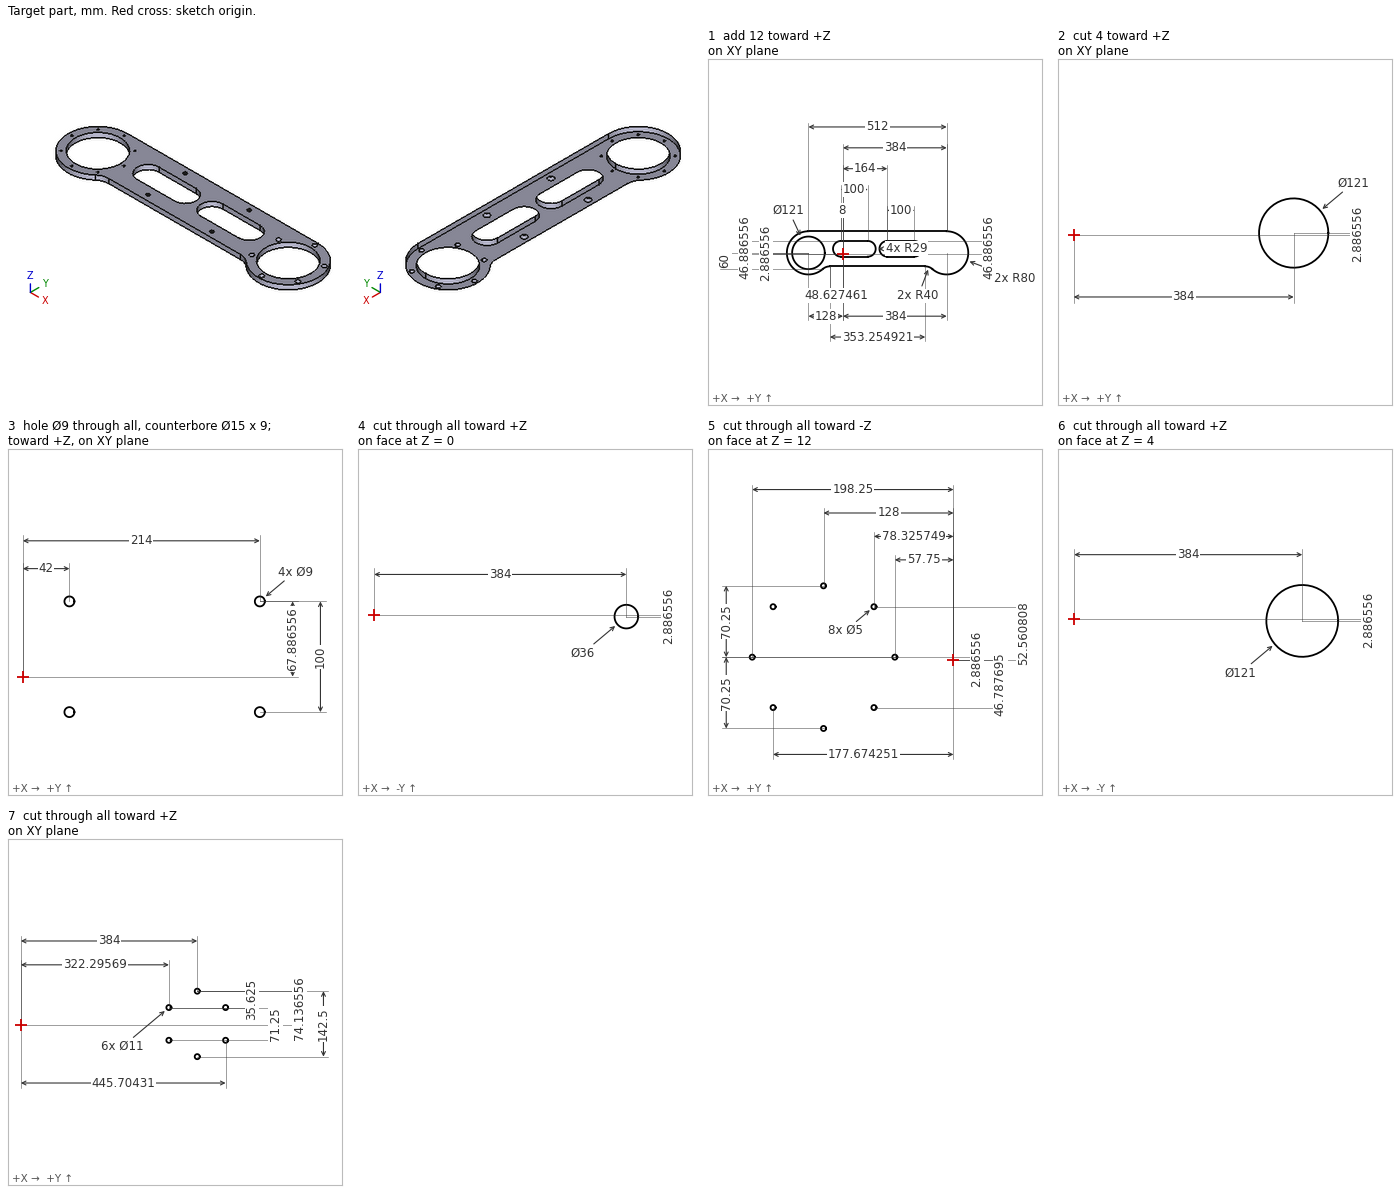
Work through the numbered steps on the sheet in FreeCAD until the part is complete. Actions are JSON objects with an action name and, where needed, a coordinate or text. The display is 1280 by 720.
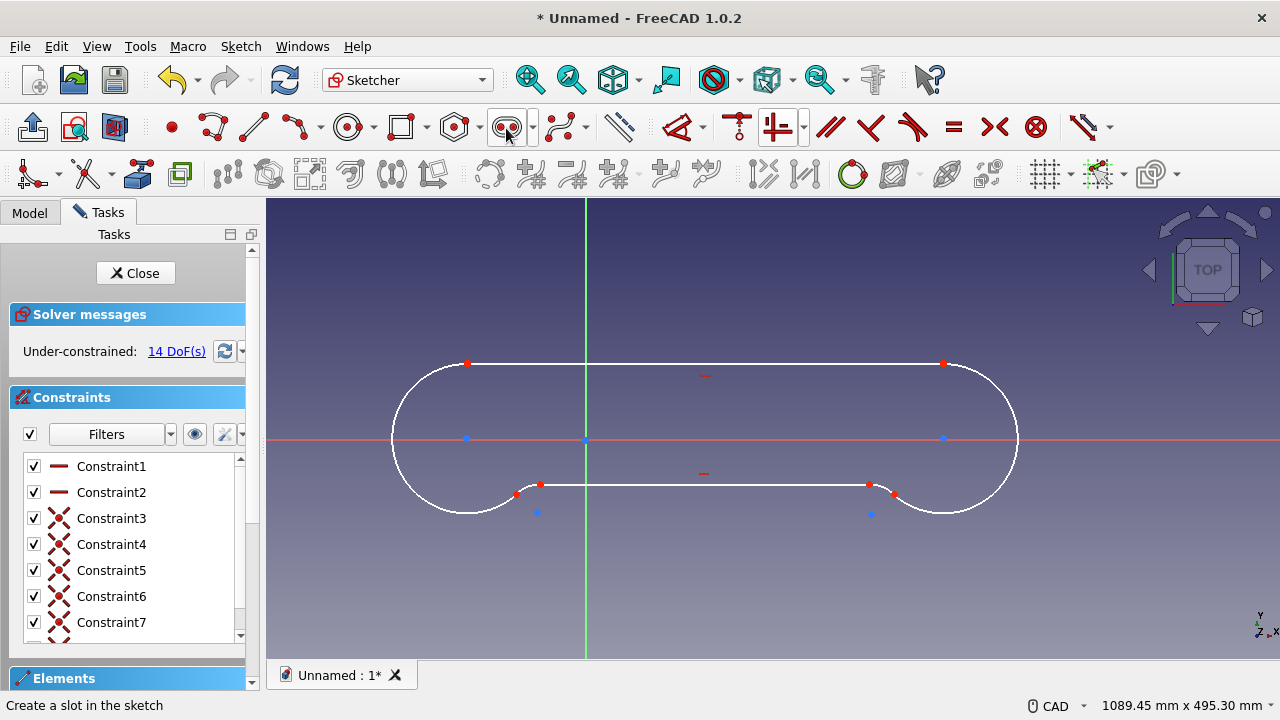
{"action": "left_click", "coordinate": [738, 424]}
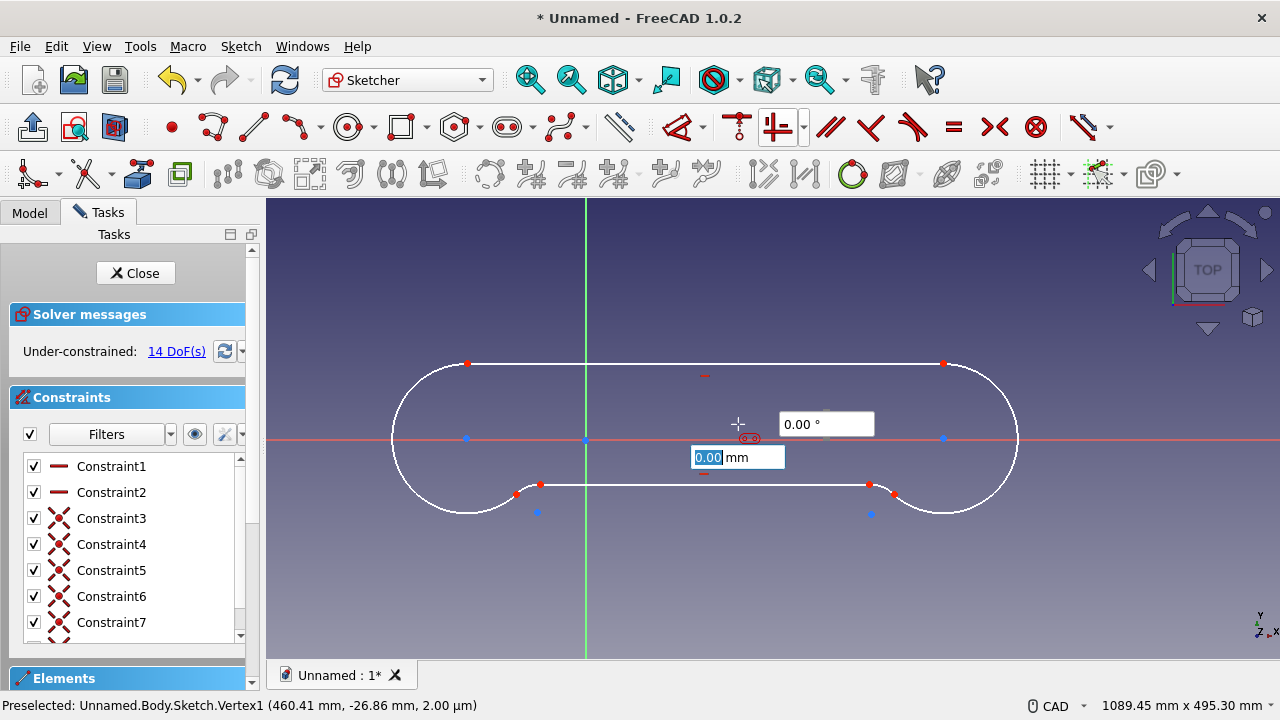
{"action": "left_click", "coordinate": [831, 424]}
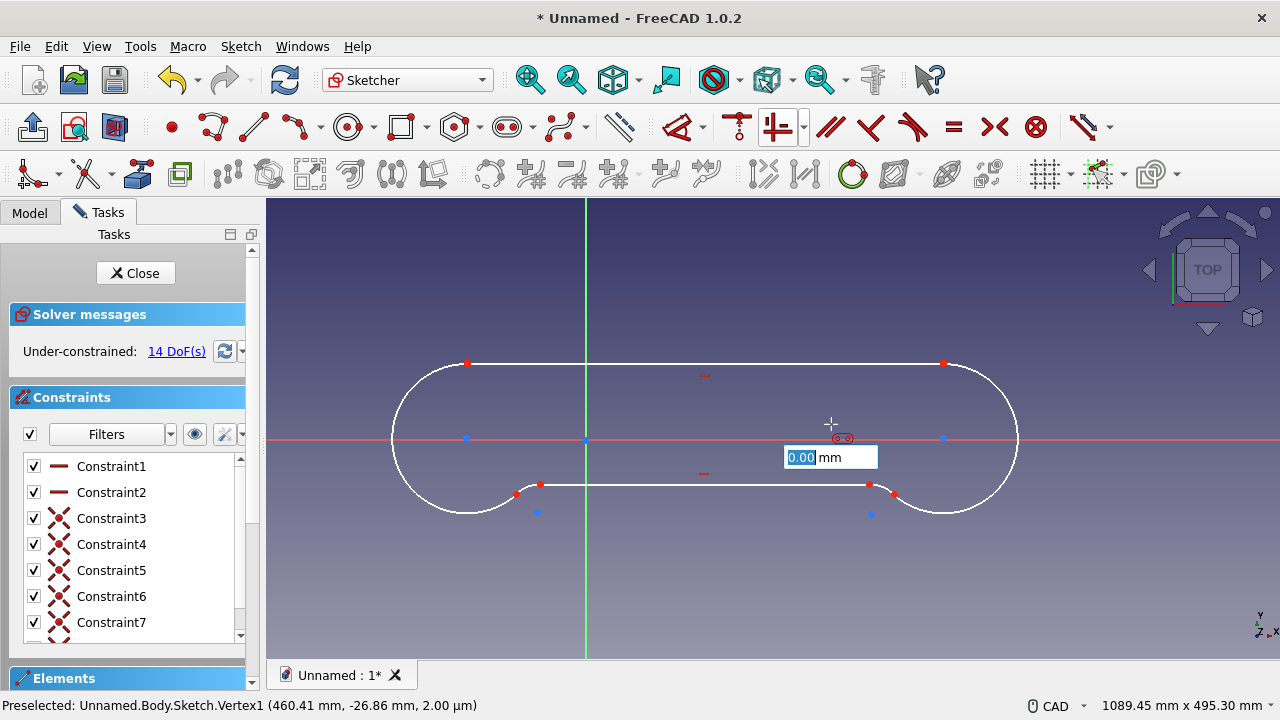
{"action": "left_click", "coordinate": [785, 397]}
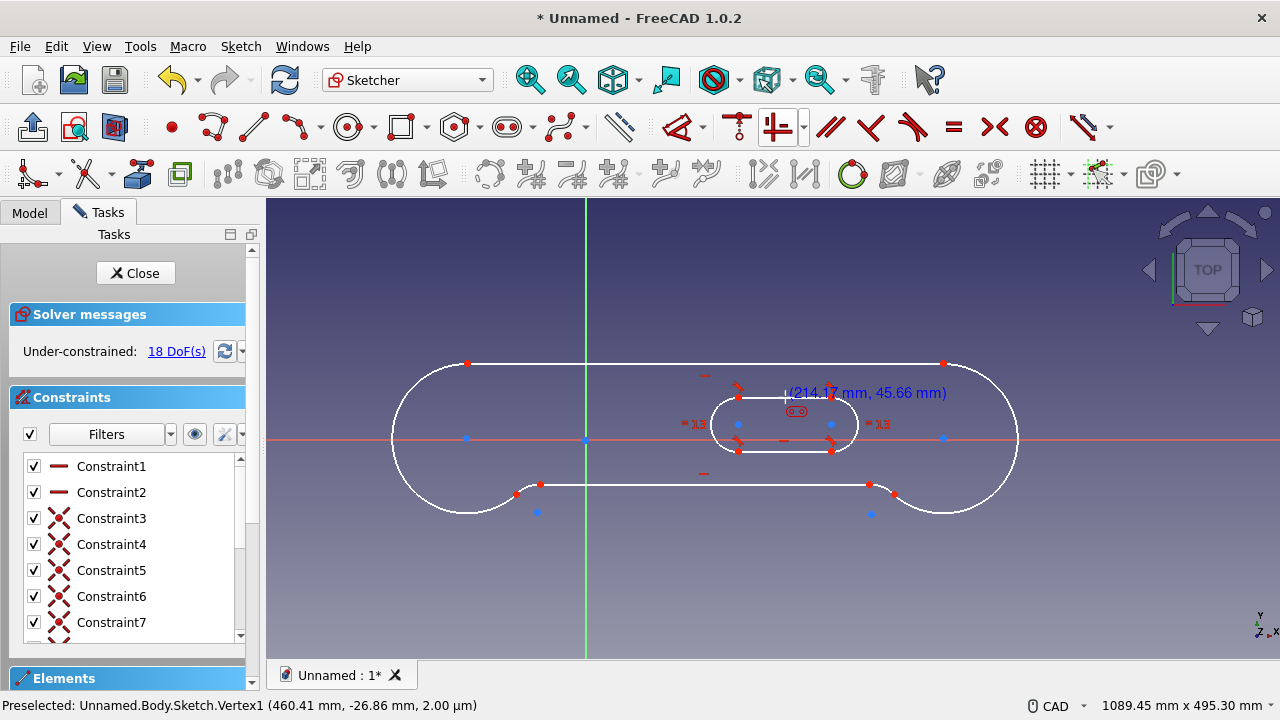
{"action": "scroll", "coordinate": [578, 424], "scroll_direction": "up", "scroll_amount": 4}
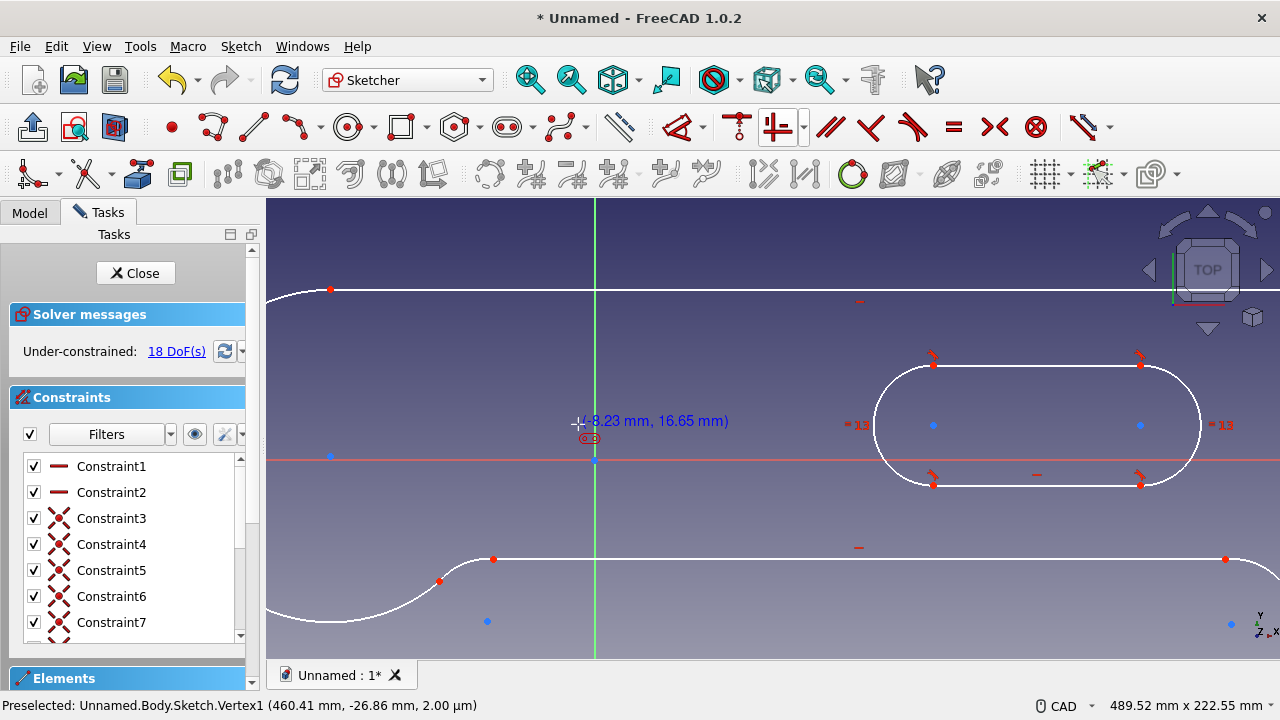
{"action": "left_click", "coordinate": [578, 423]}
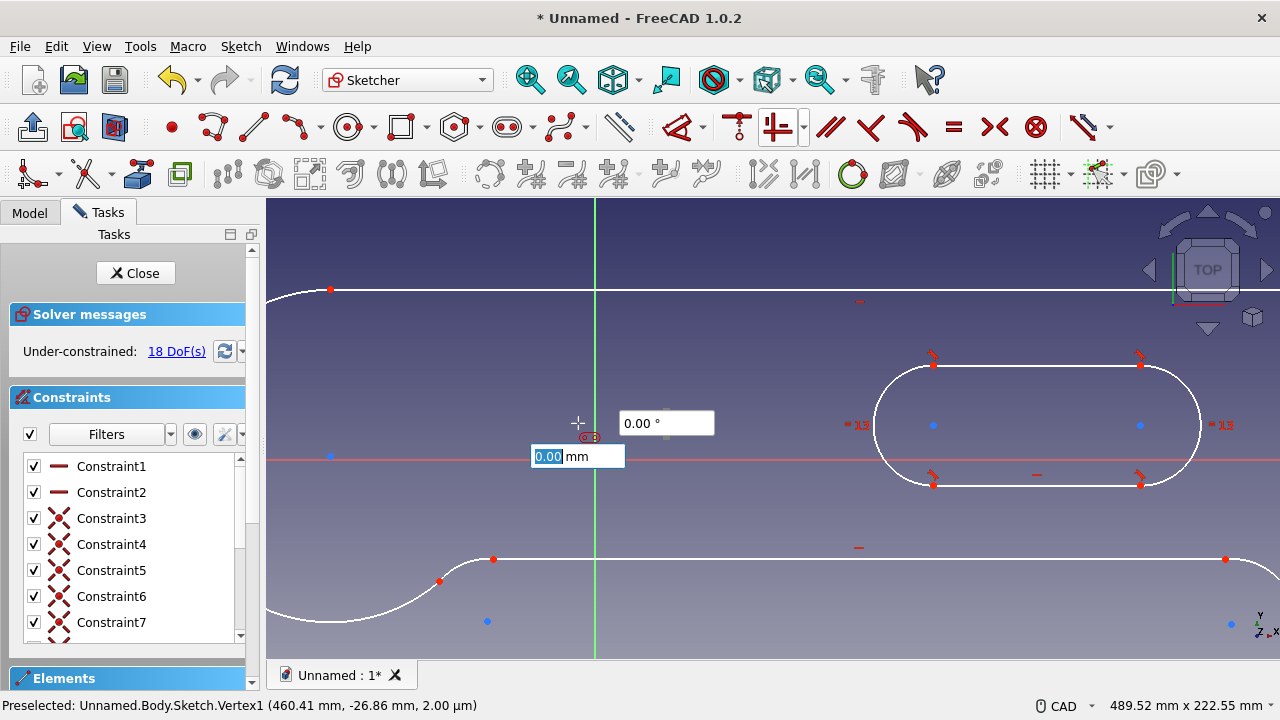
{"action": "left_click", "coordinate": [785, 423]}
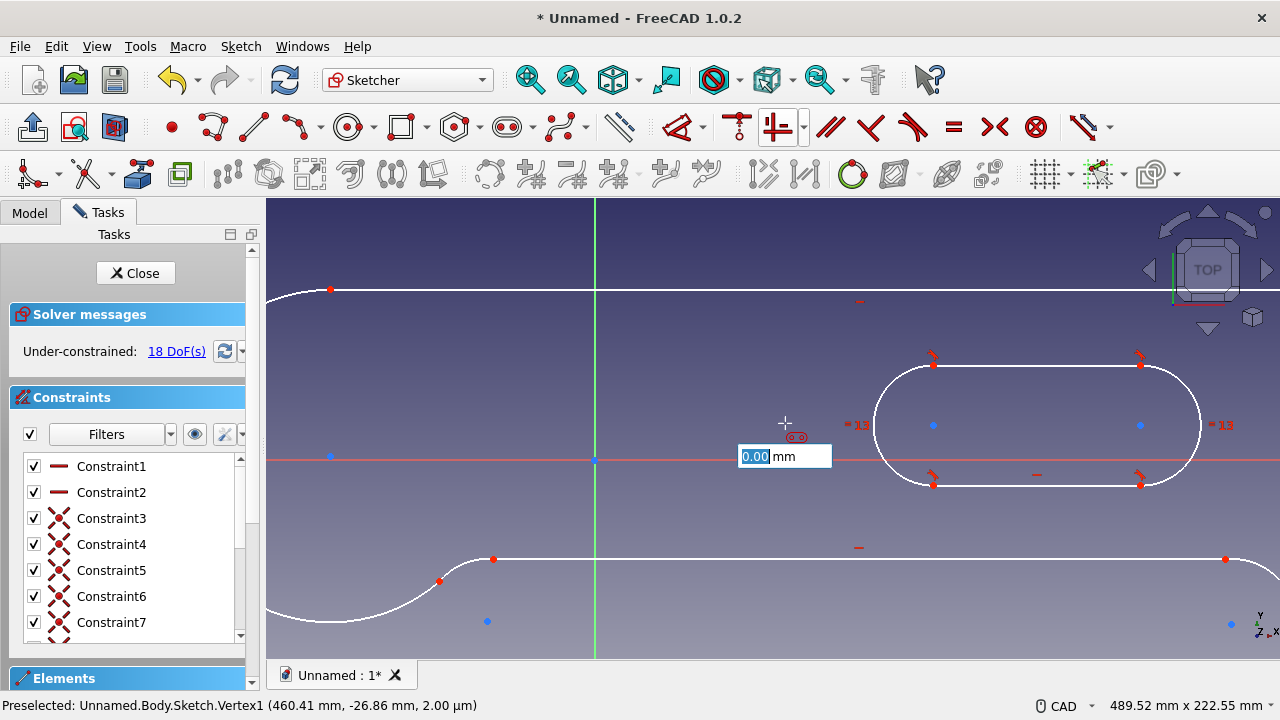
{"action": "left_click", "coordinate": [682, 363]}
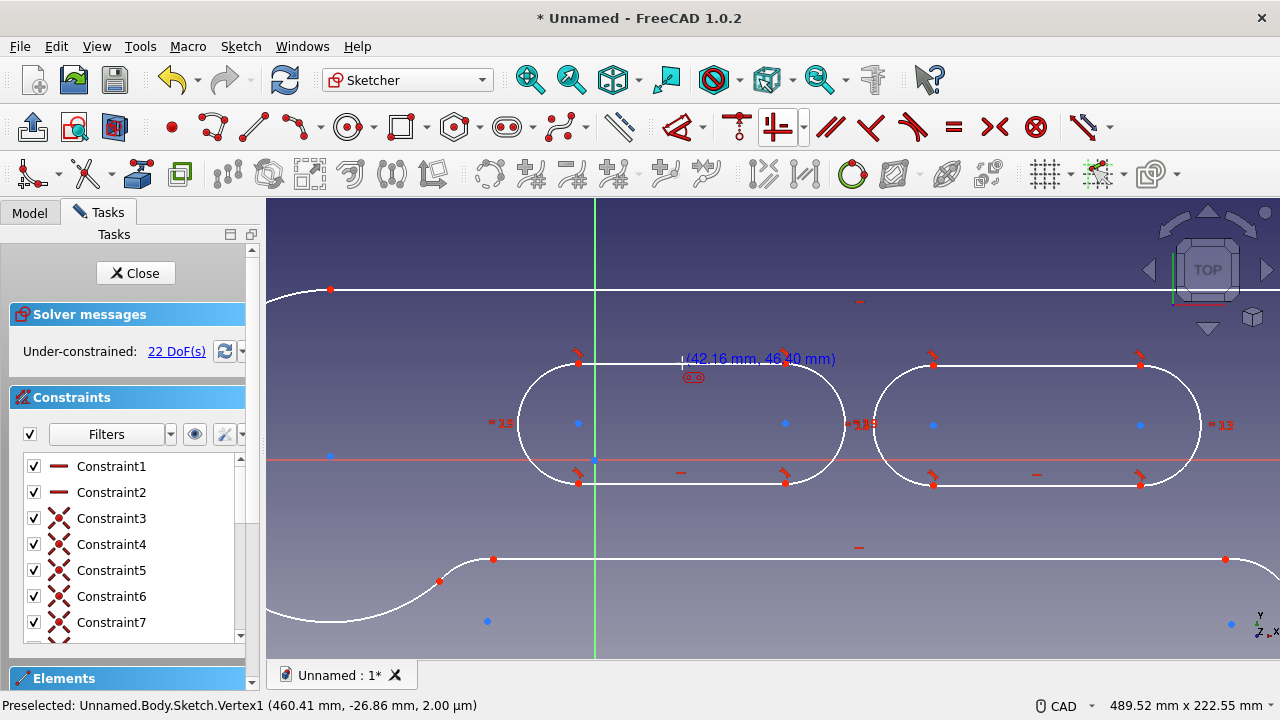
{"action": "left_click", "coordinate": [348, 128]}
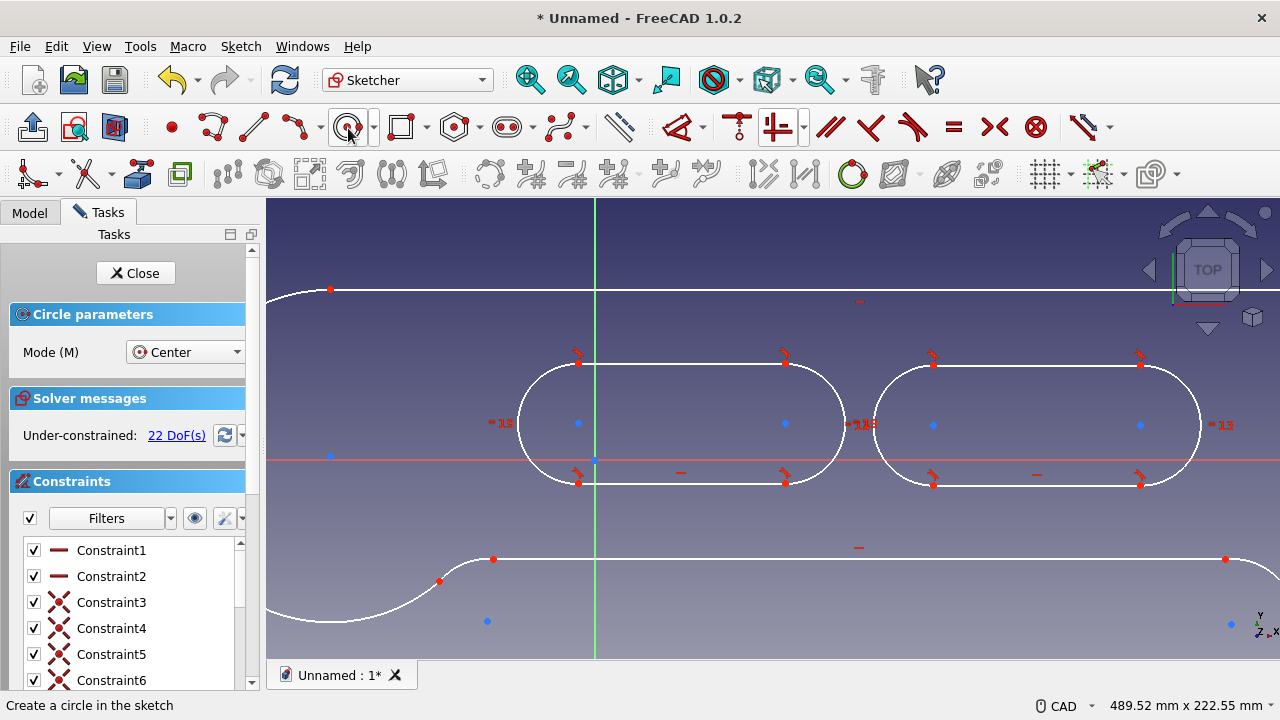
{"action": "scroll", "coordinate": [330, 454], "scroll_direction": "up", "scroll_amount": 5}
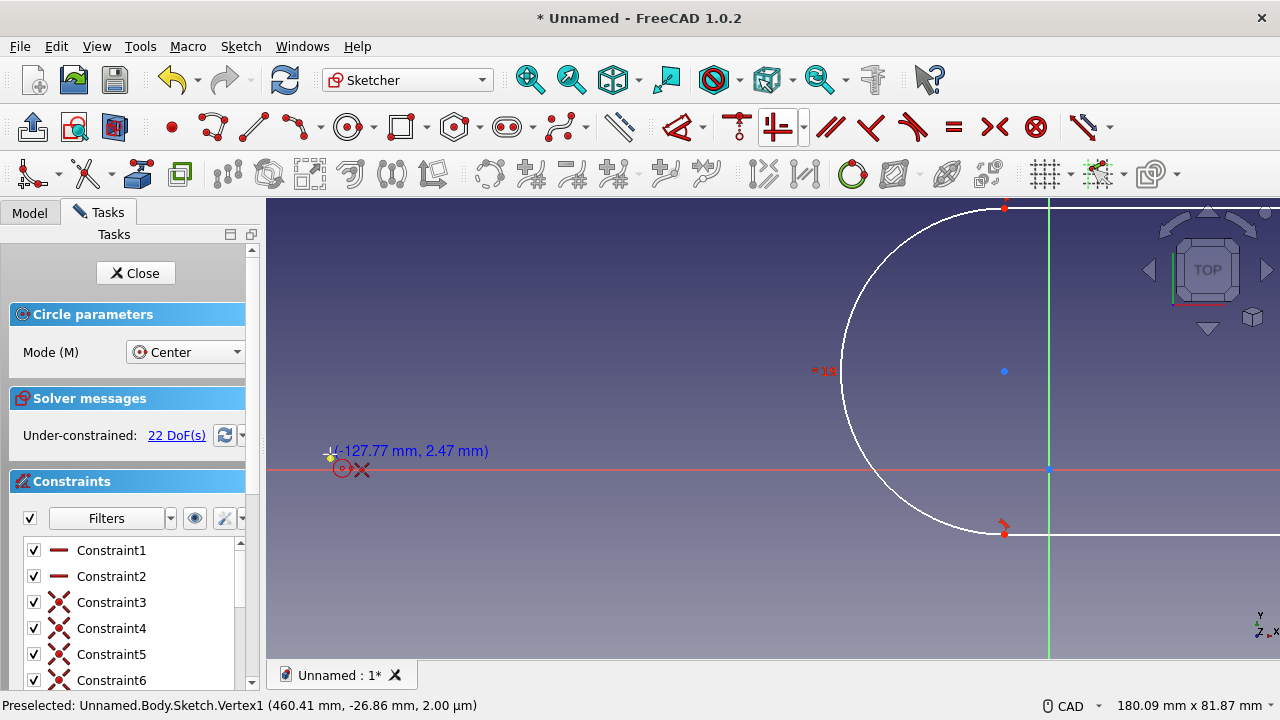
{"action": "left_click", "coordinate": [329, 453]}